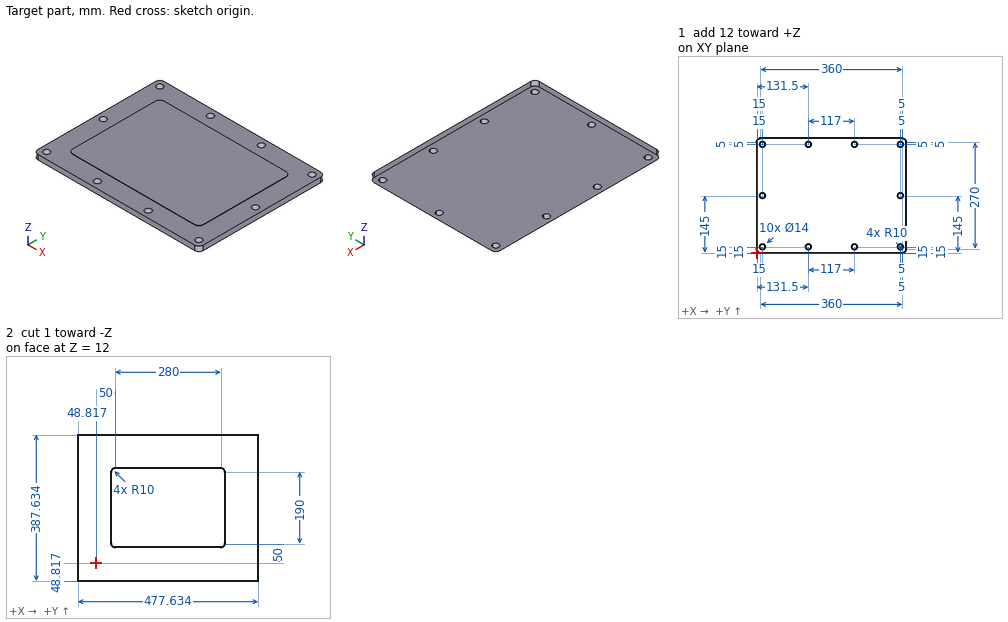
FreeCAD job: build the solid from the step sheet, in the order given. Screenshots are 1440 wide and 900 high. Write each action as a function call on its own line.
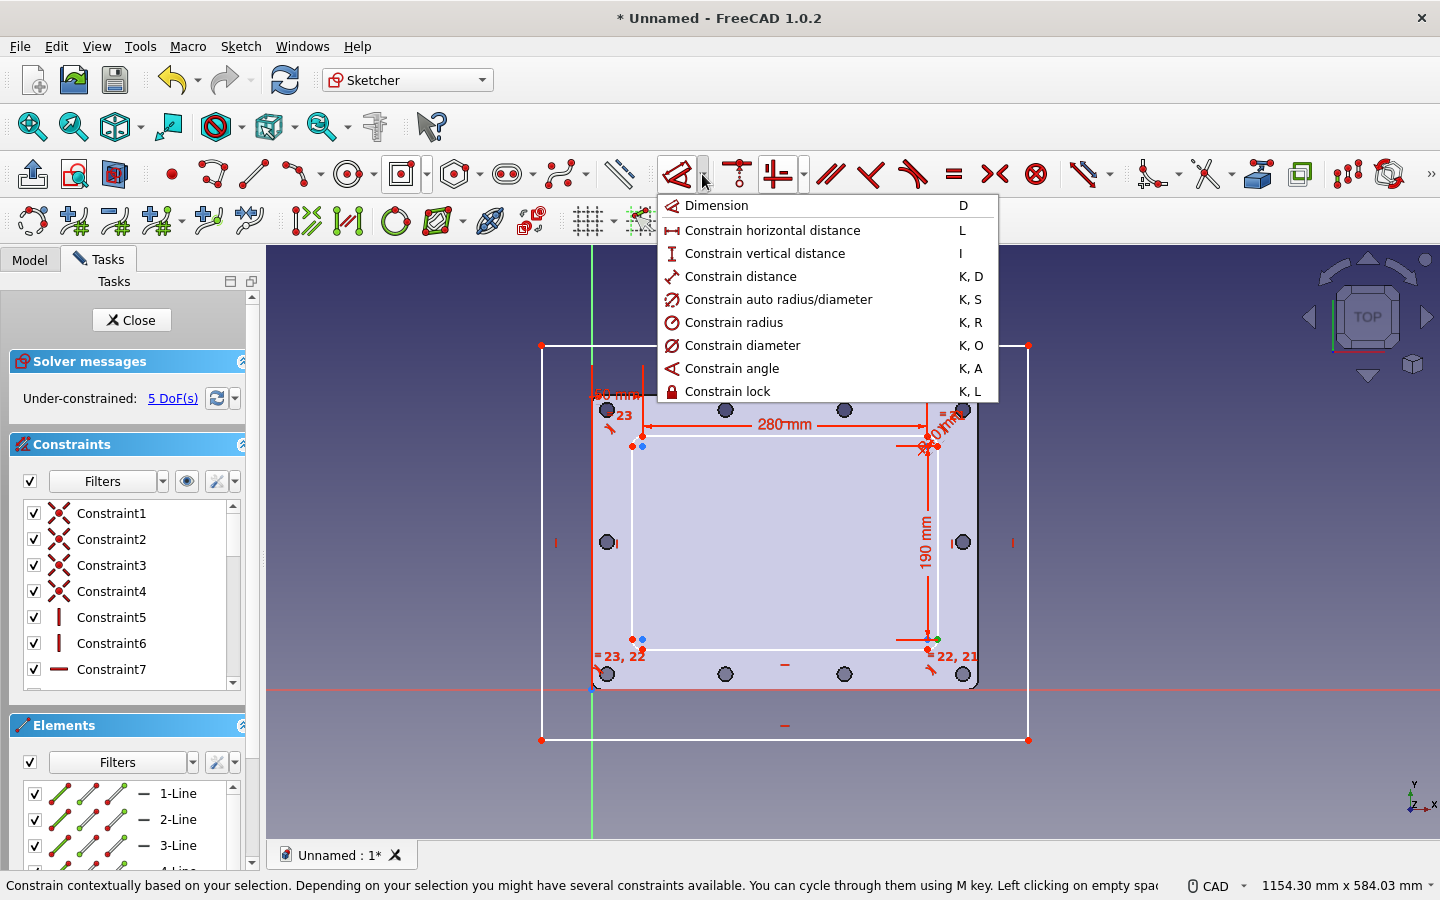
click(828, 254)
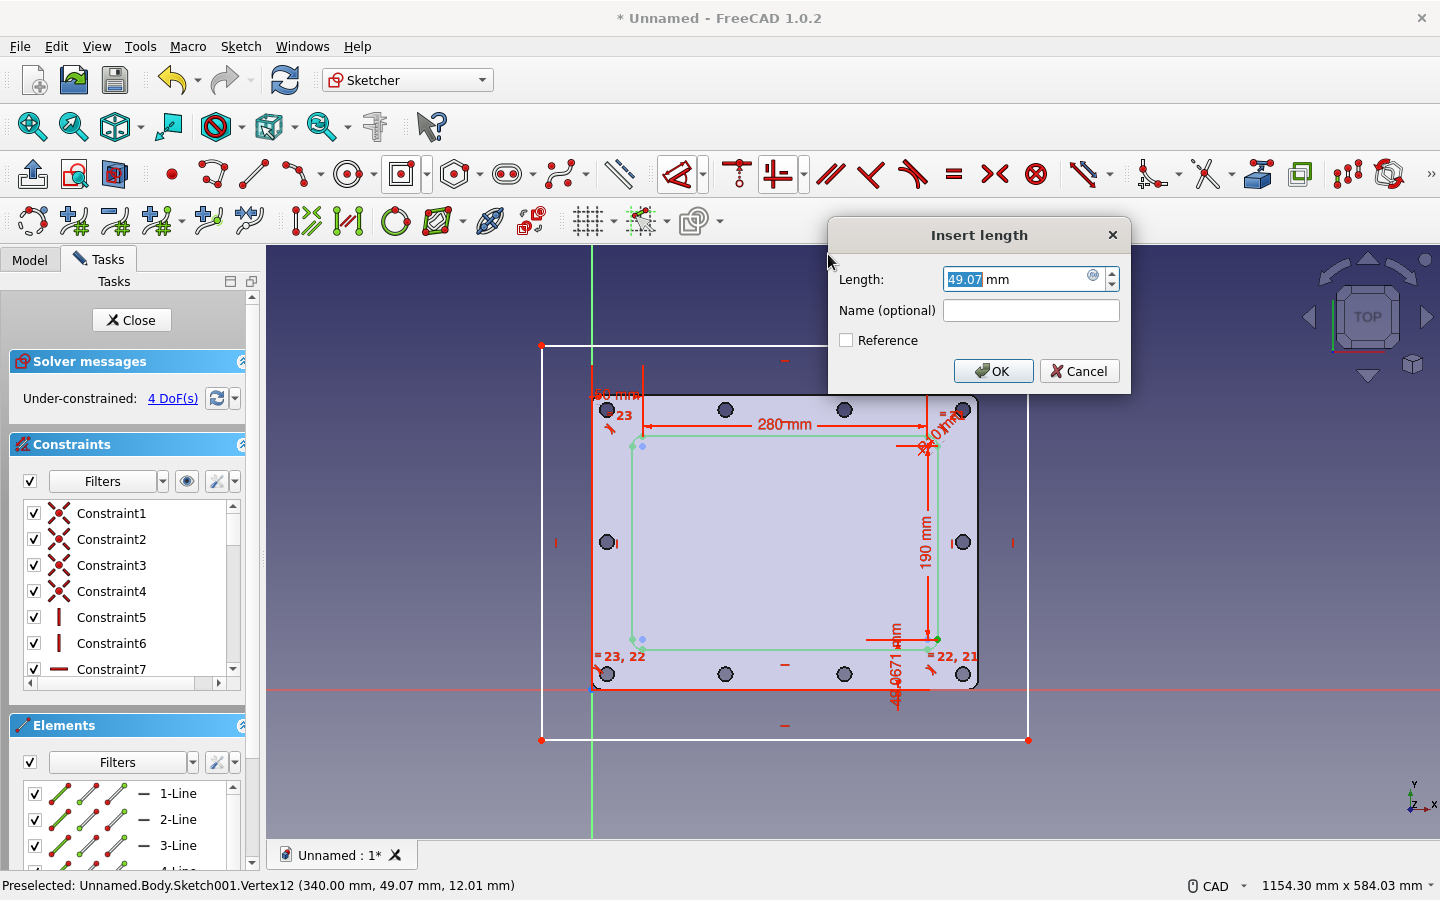
text(50)
key(Return)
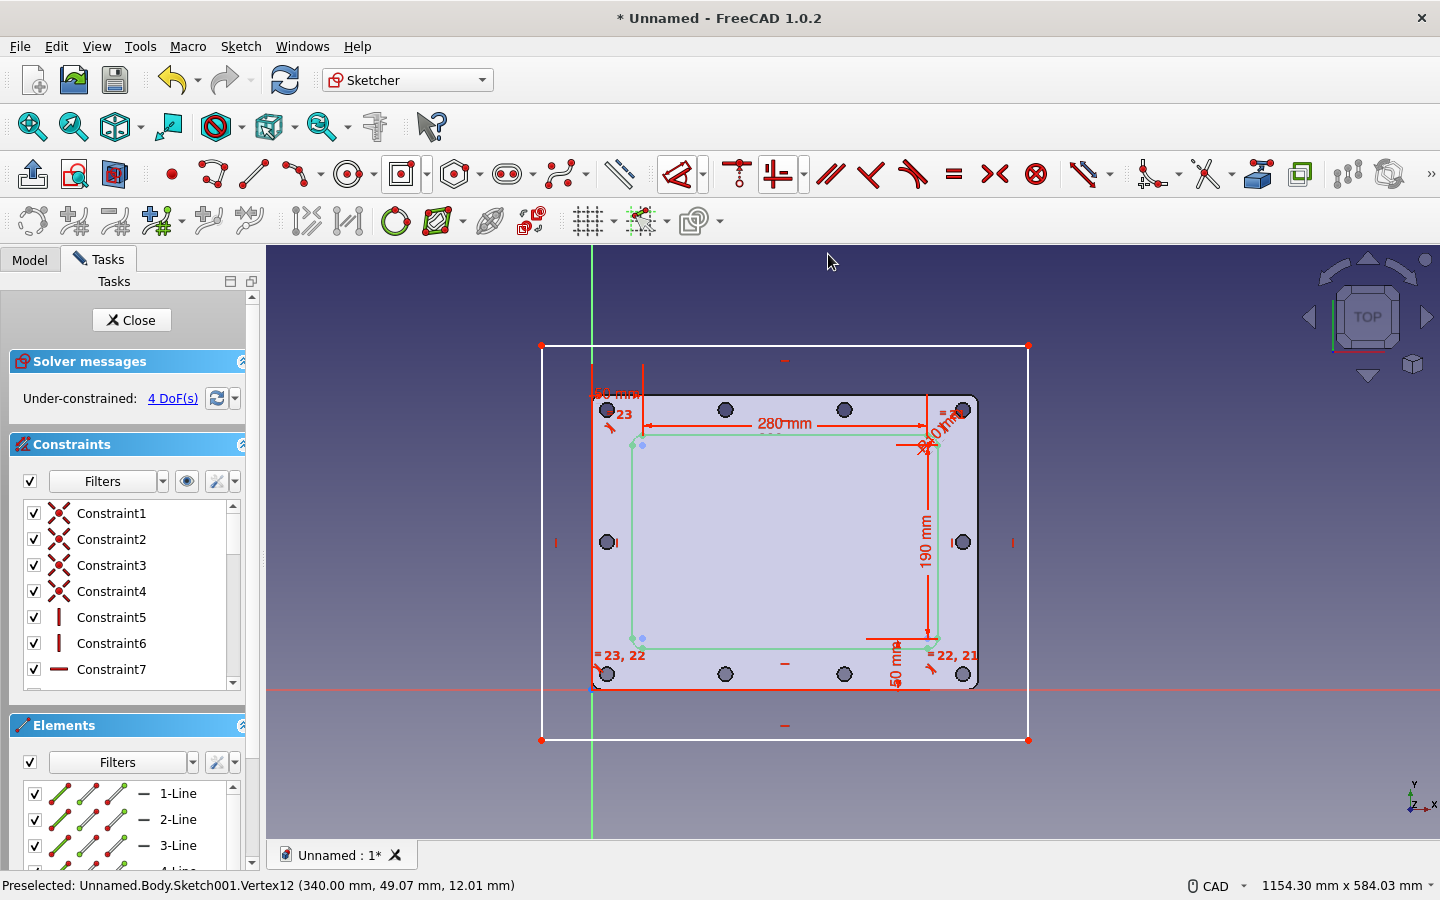
click(542, 464)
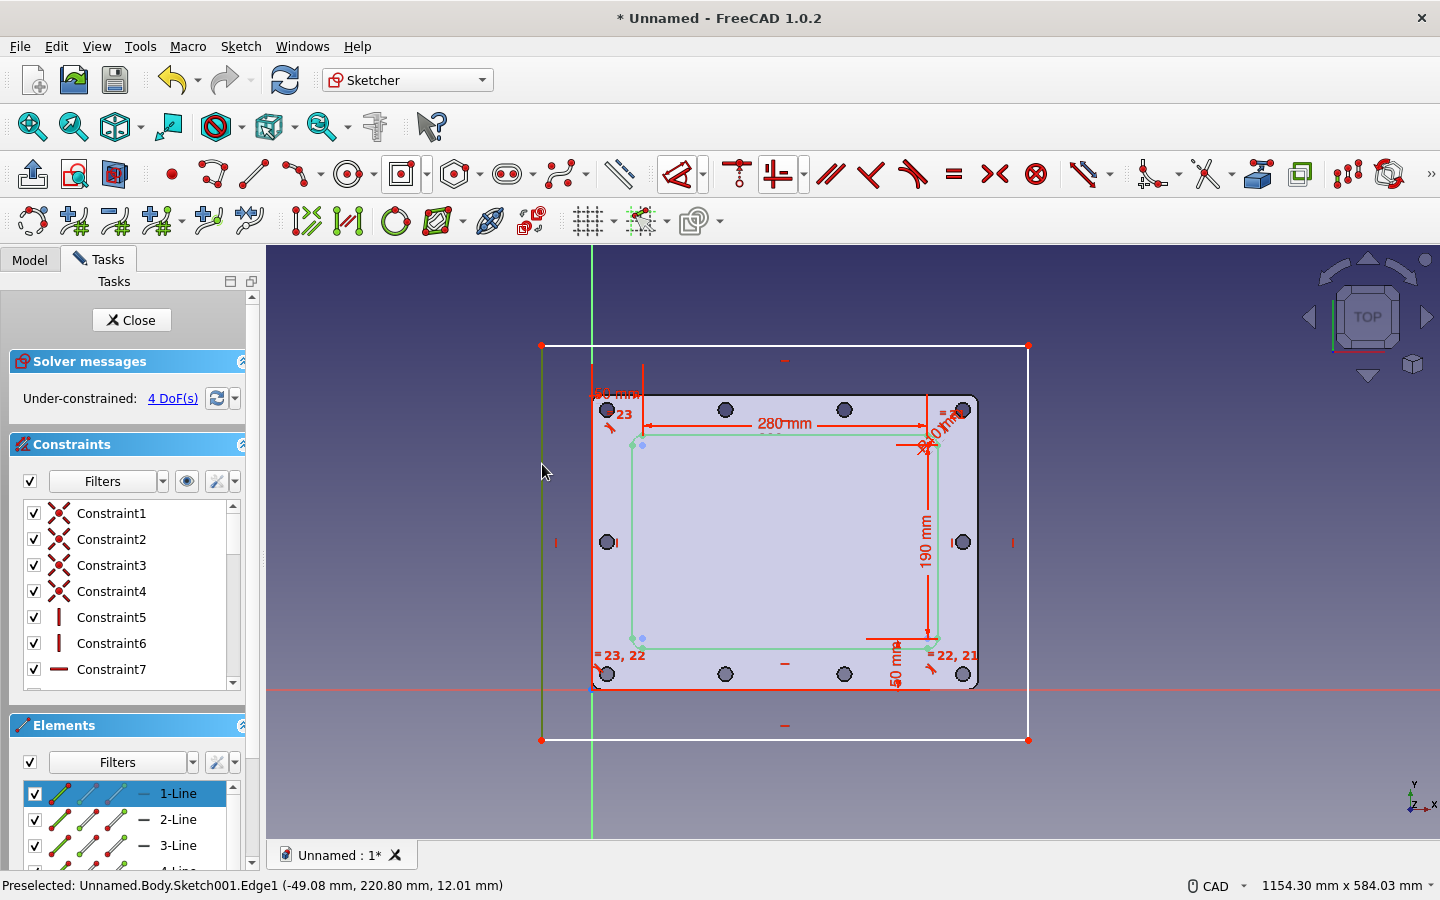
key(i)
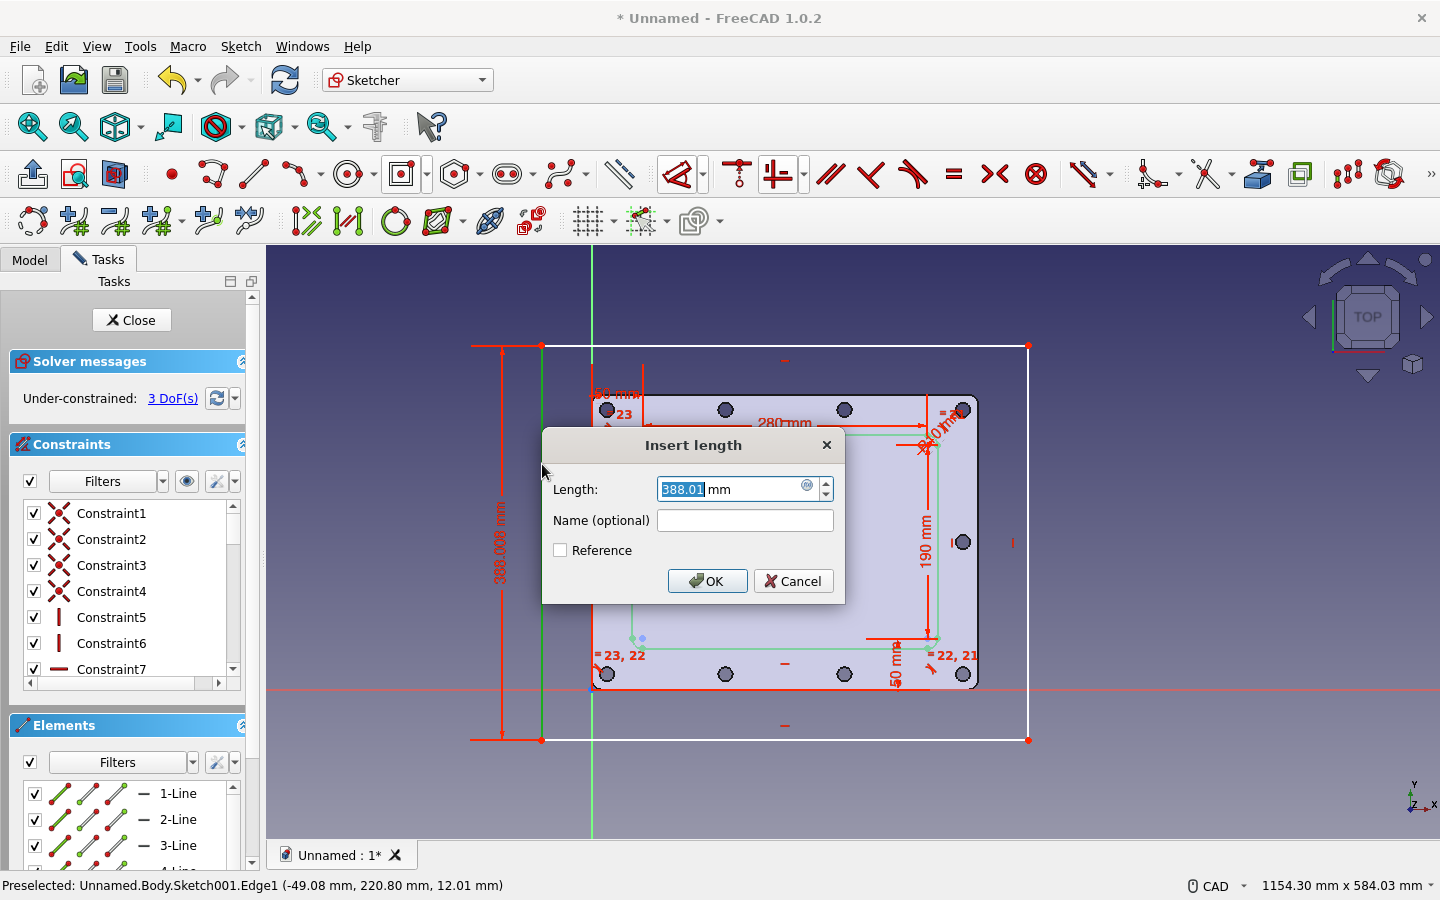
text(387.634)
key(Return)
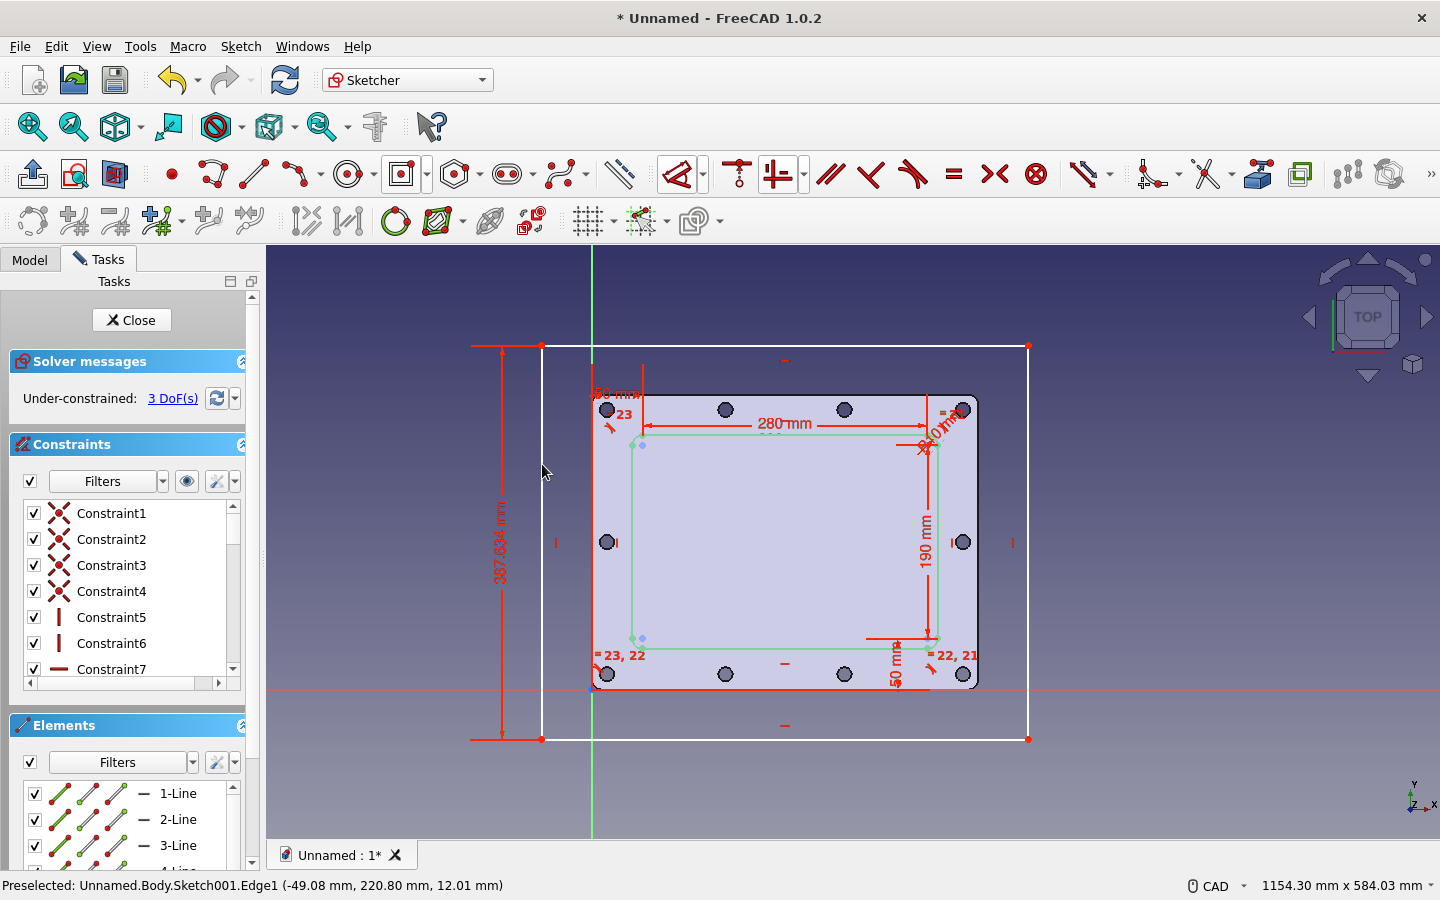
click(688, 740)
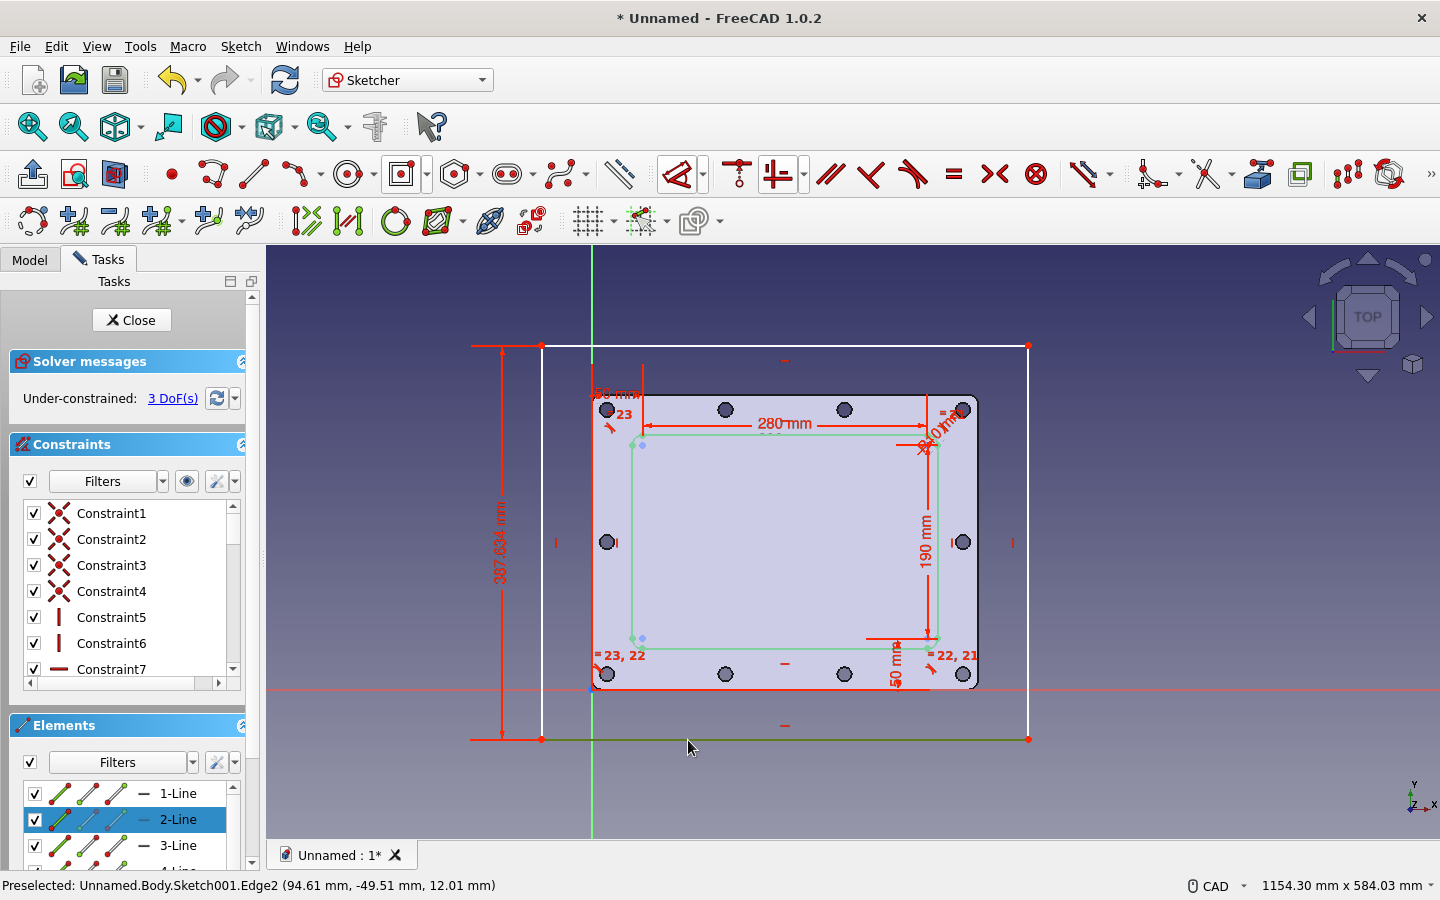
click(702, 174)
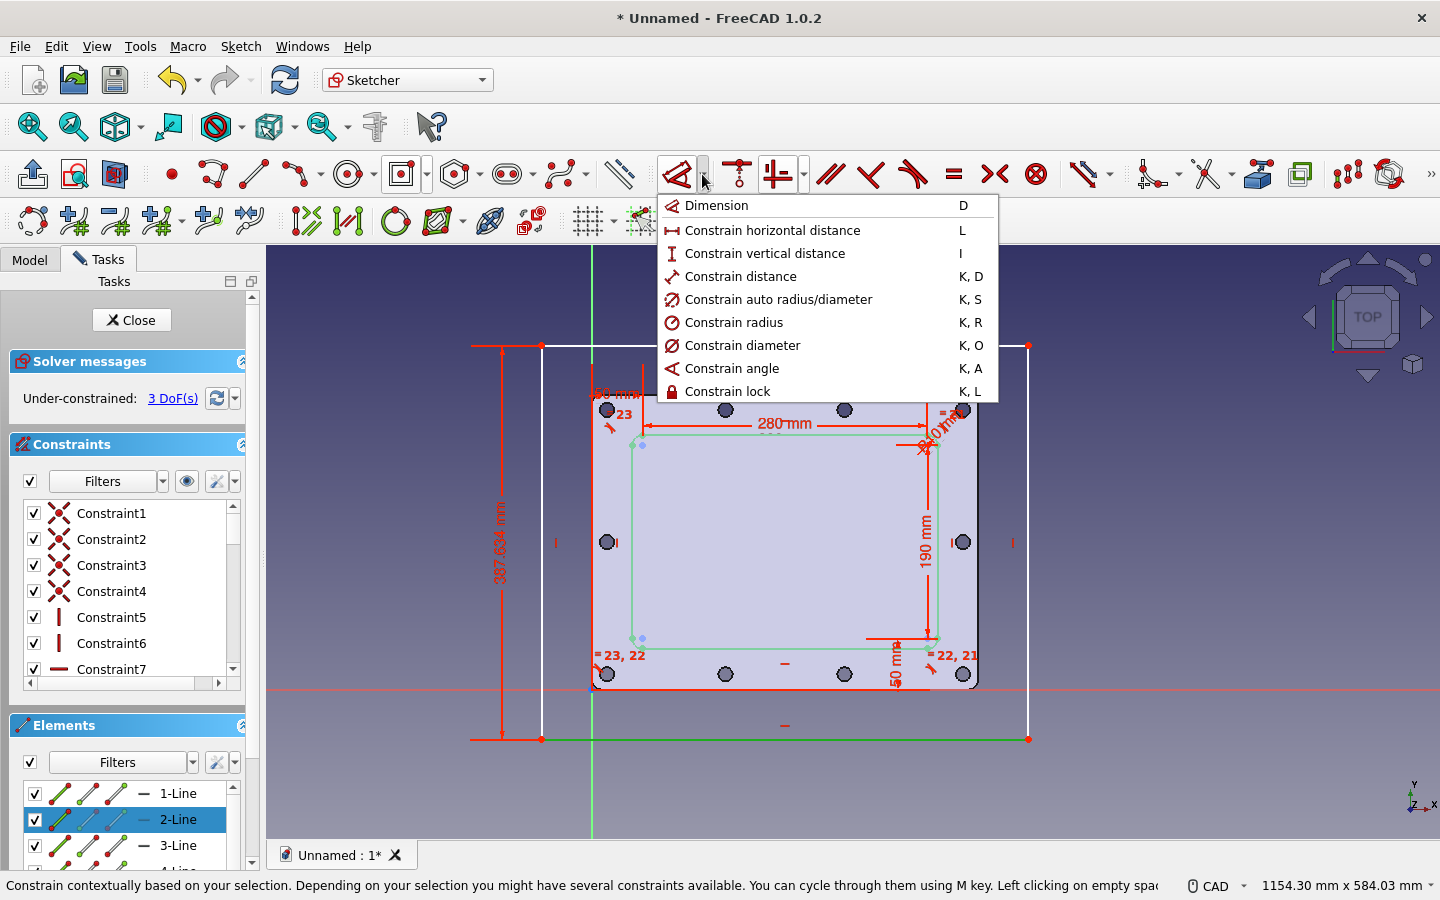
click(828, 230)